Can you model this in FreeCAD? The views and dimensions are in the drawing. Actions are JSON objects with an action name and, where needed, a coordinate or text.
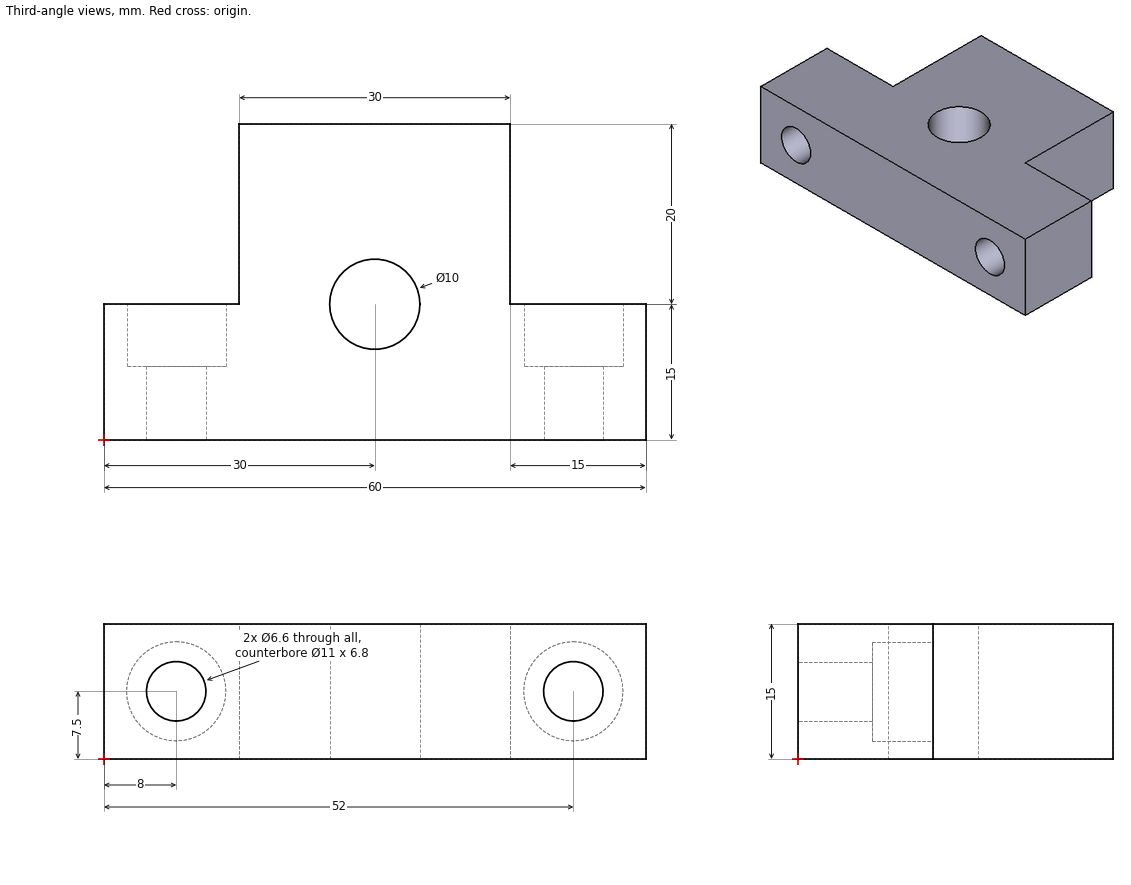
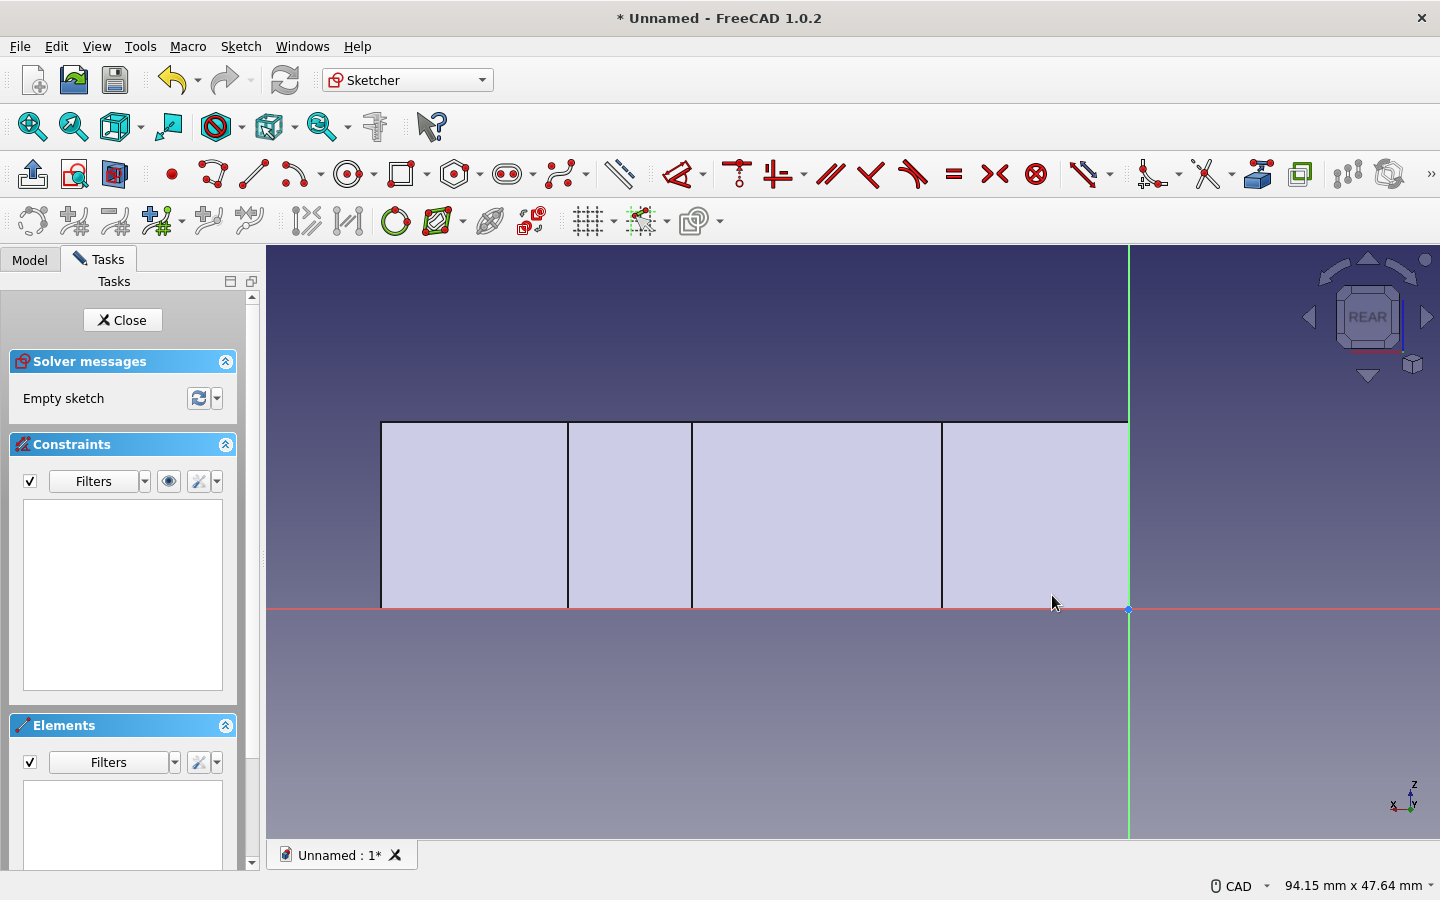
{"action": "left_click", "coordinate": [348, 174]}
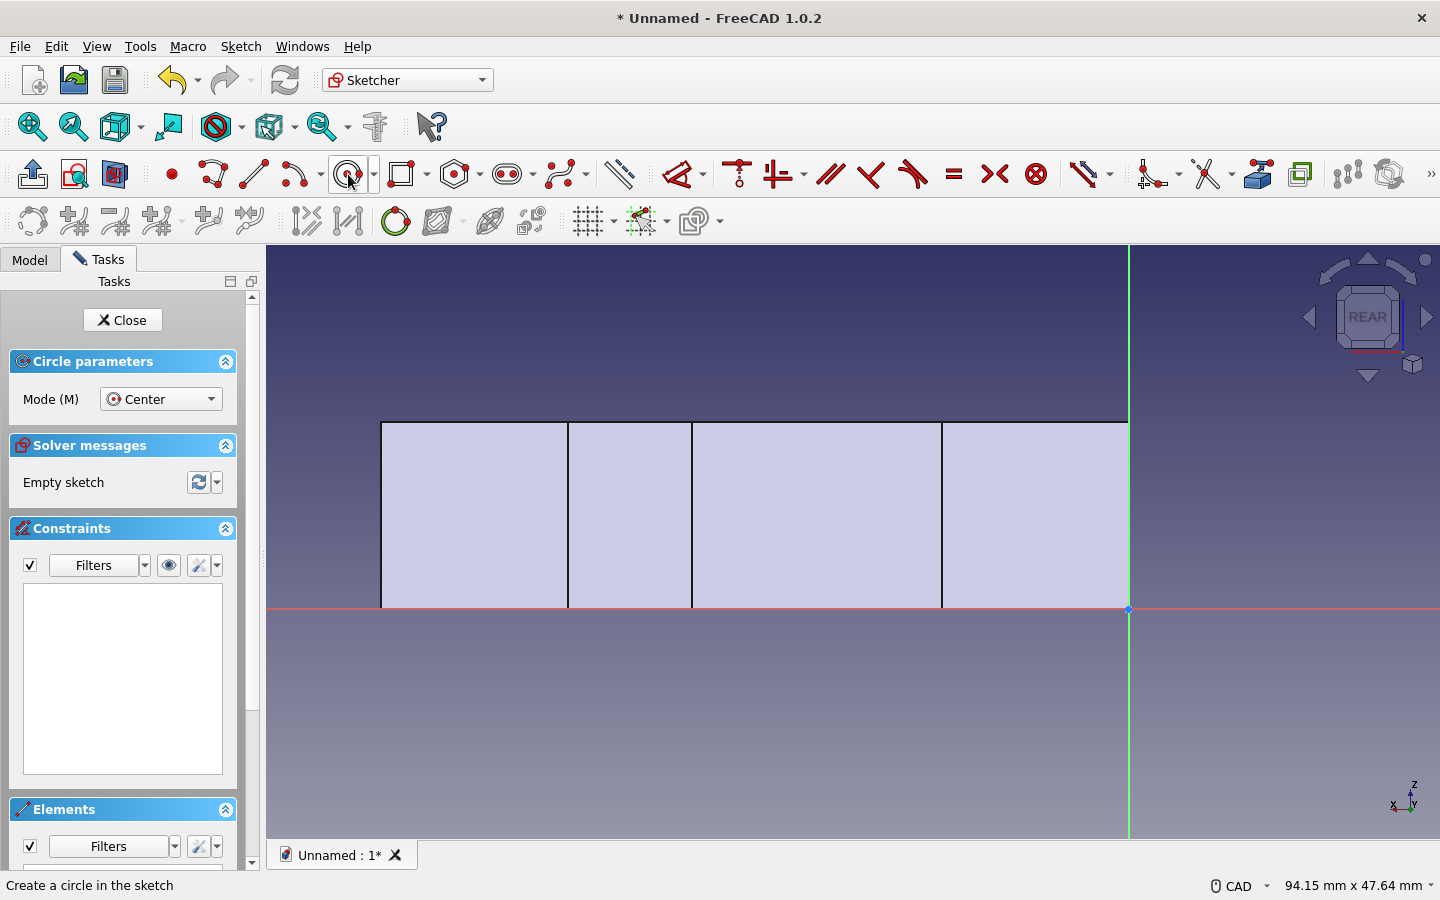
{"action": "left_click", "coordinate": [1029, 516]}
{"action": "left_click", "coordinate": [1058, 487]}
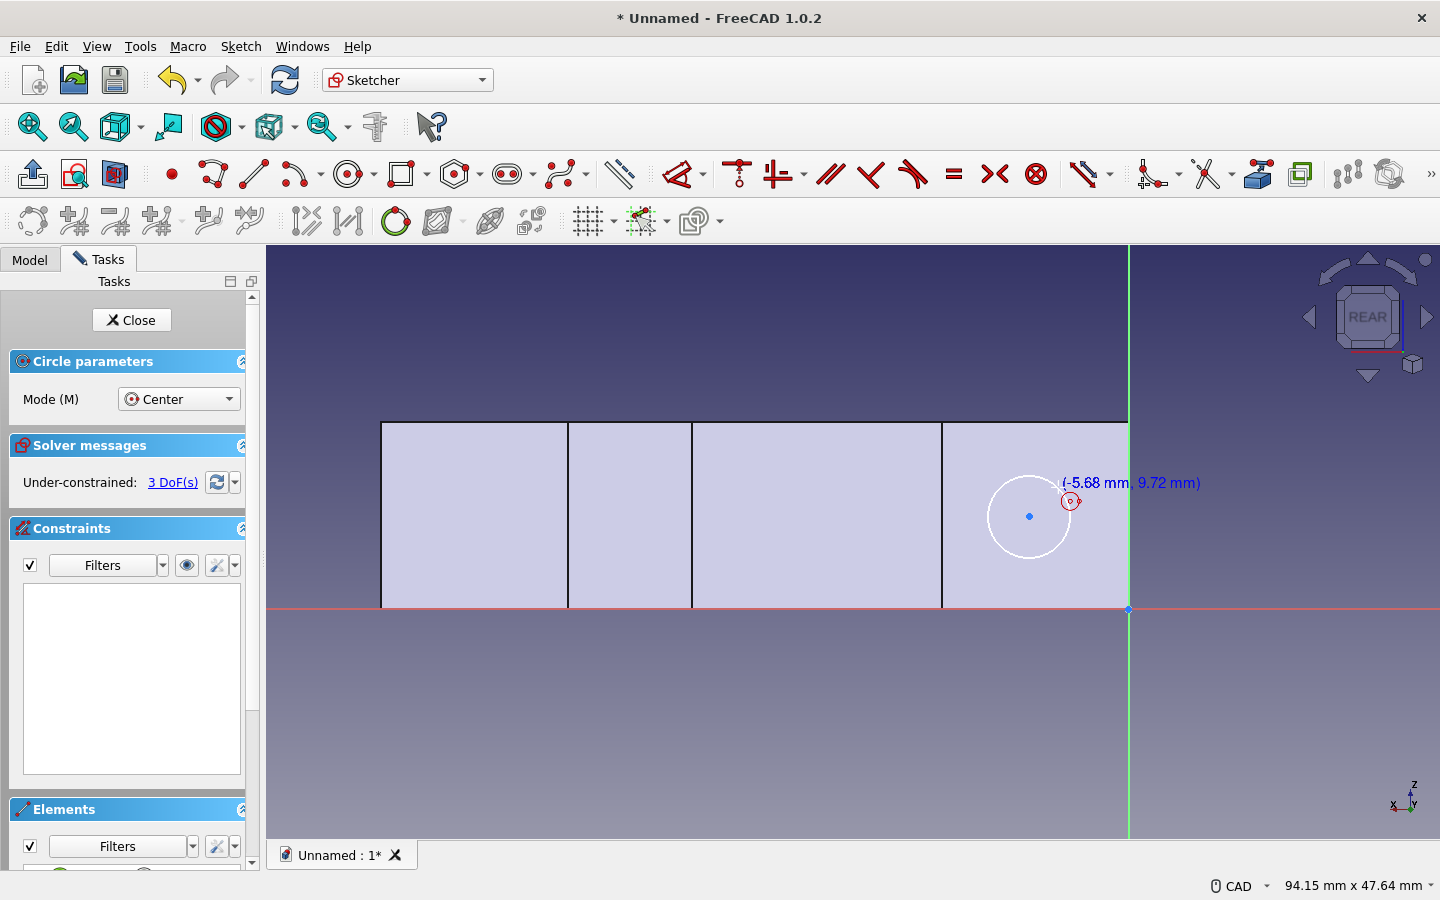
{"action": "left_click", "coordinate": [480, 516]}
{"action": "left_click", "coordinate": [510, 487]}
{"action": "key", "text": "Escape"}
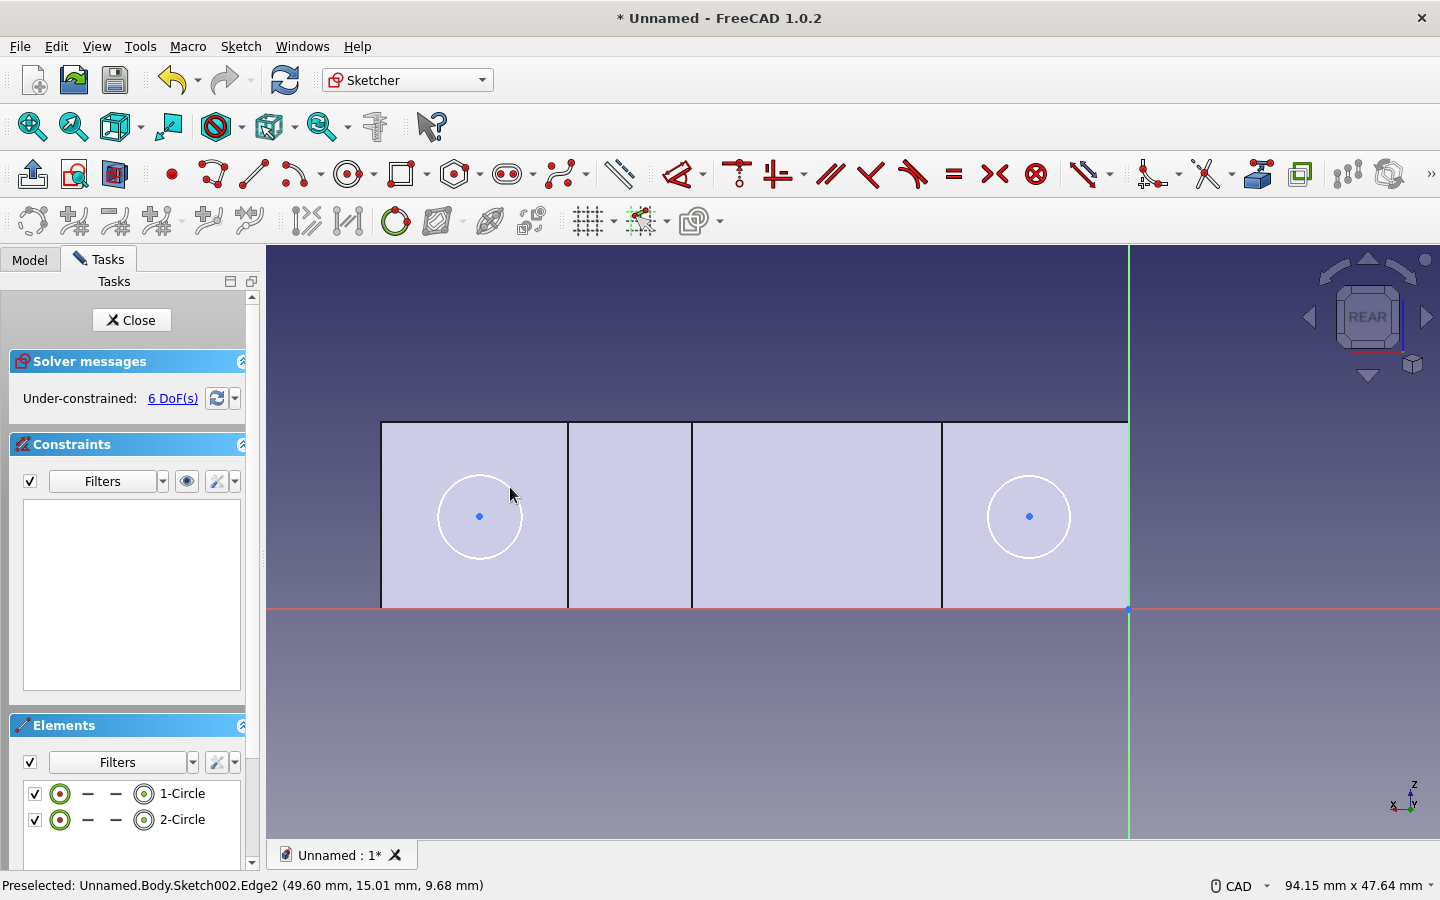
{"action": "left_click", "coordinate": [1058, 488]}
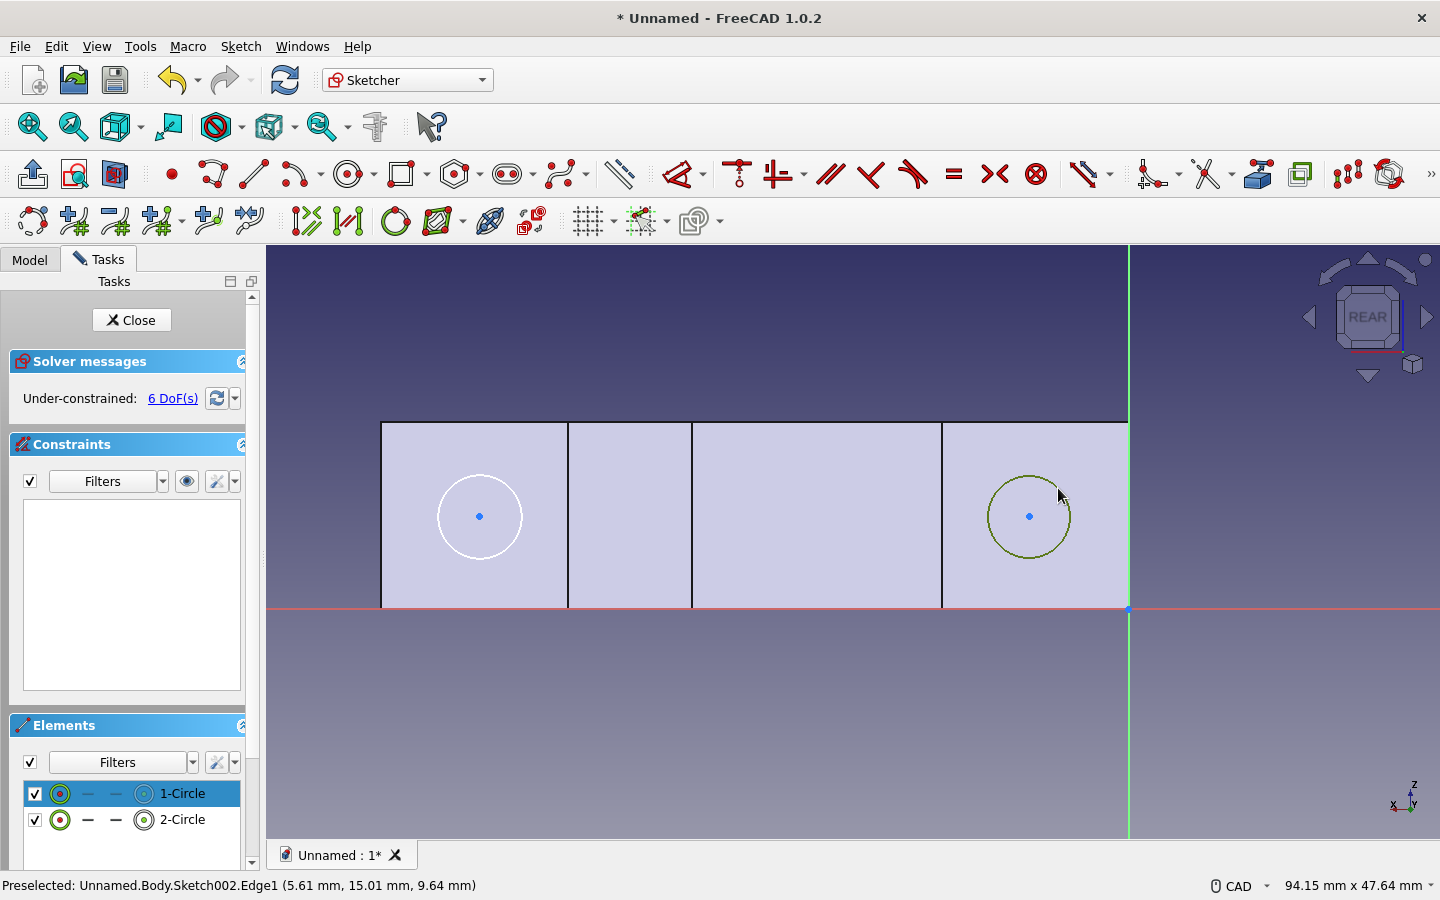
{"action": "left_click", "coordinate": [509, 487]}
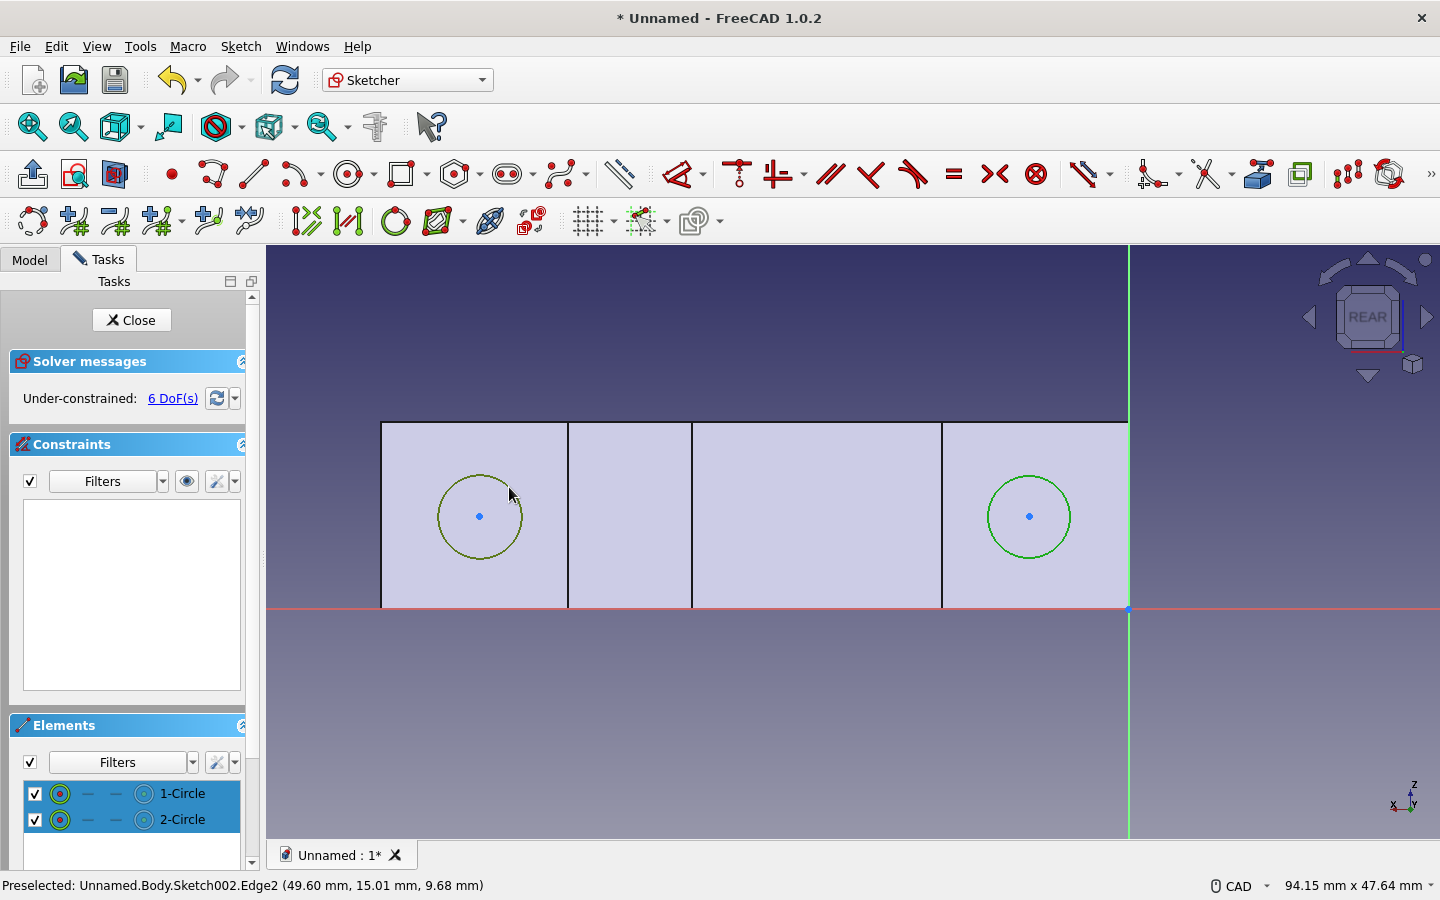
{"action": "left_click", "coordinate": [954, 174]}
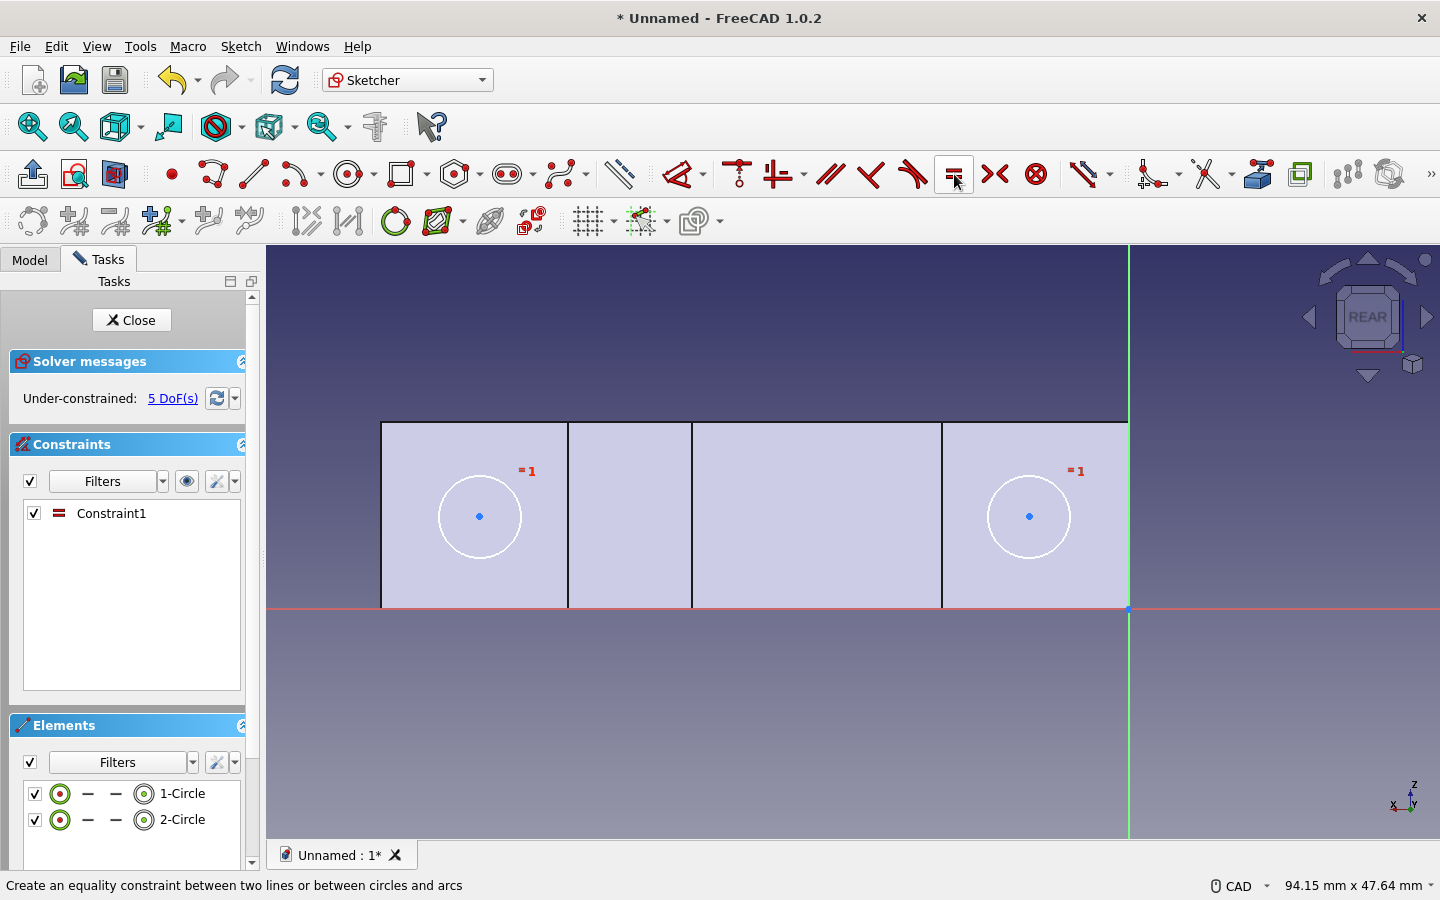
{"action": "left_click", "coordinate": [1029, 517]}